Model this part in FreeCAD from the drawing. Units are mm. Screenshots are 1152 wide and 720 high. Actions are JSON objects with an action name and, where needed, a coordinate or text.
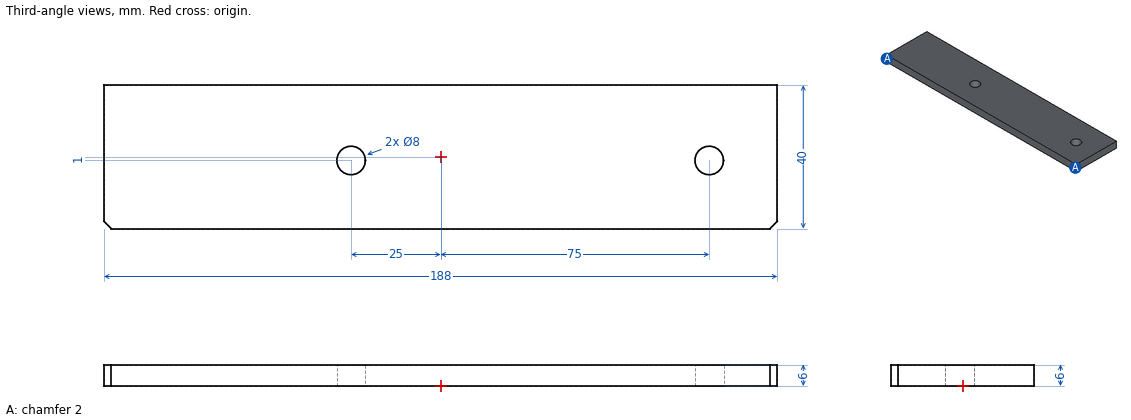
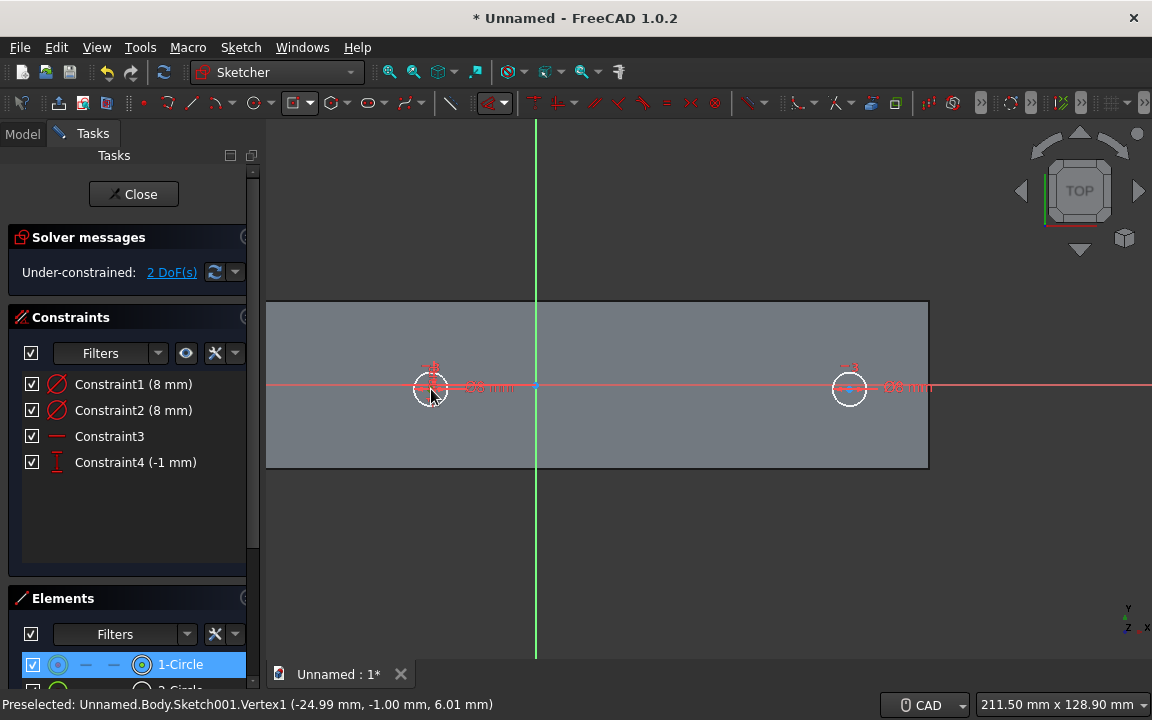
{"action": "left_click", "coordinate": [506, 104]}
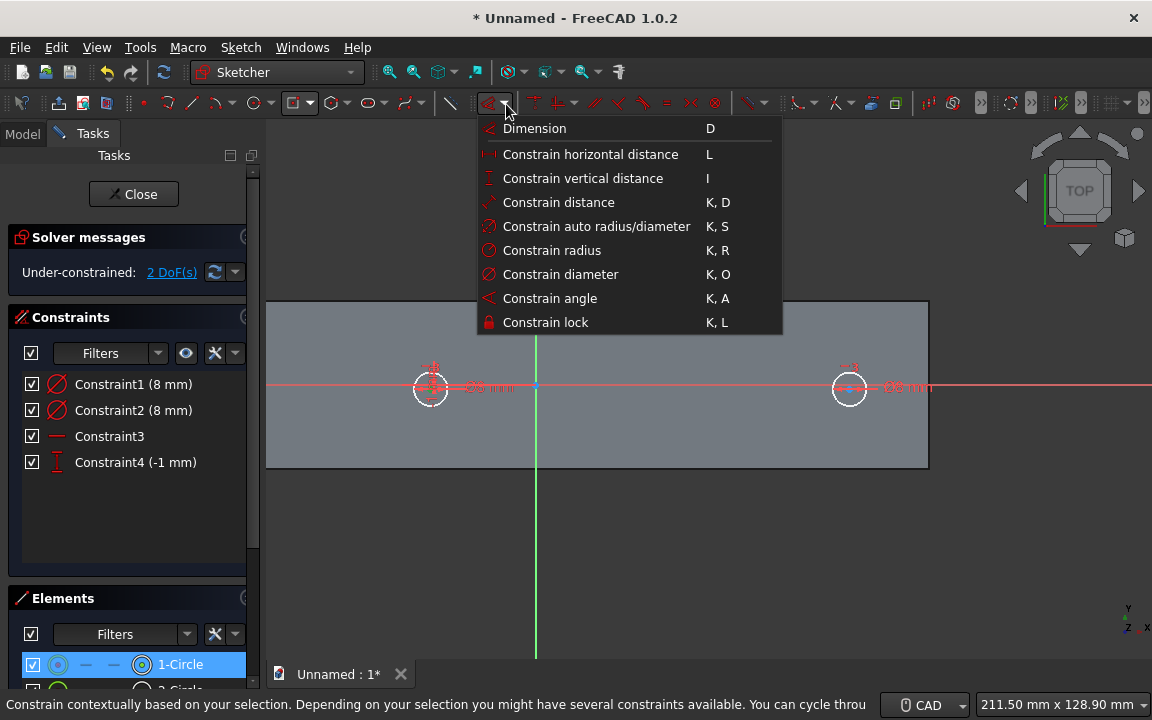
{"action": "left_click", "coordinate": [630, 154]}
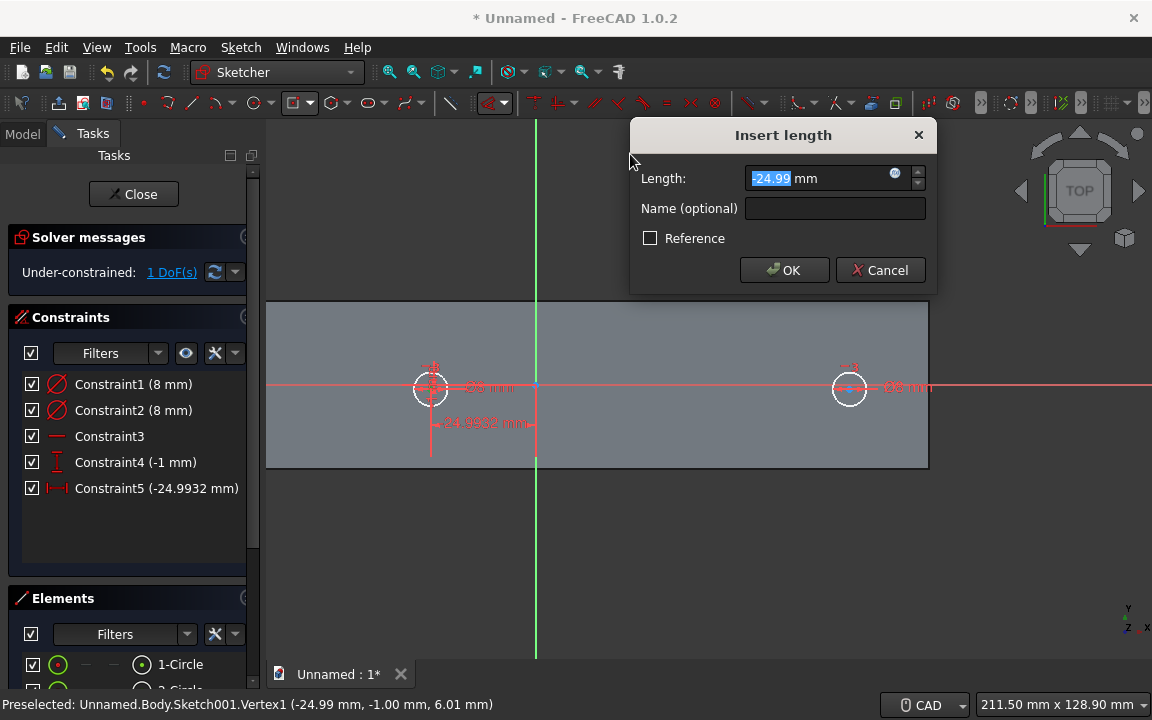
{"action": "type", "text": "-25"}
{"action": "key", "text": "Return"}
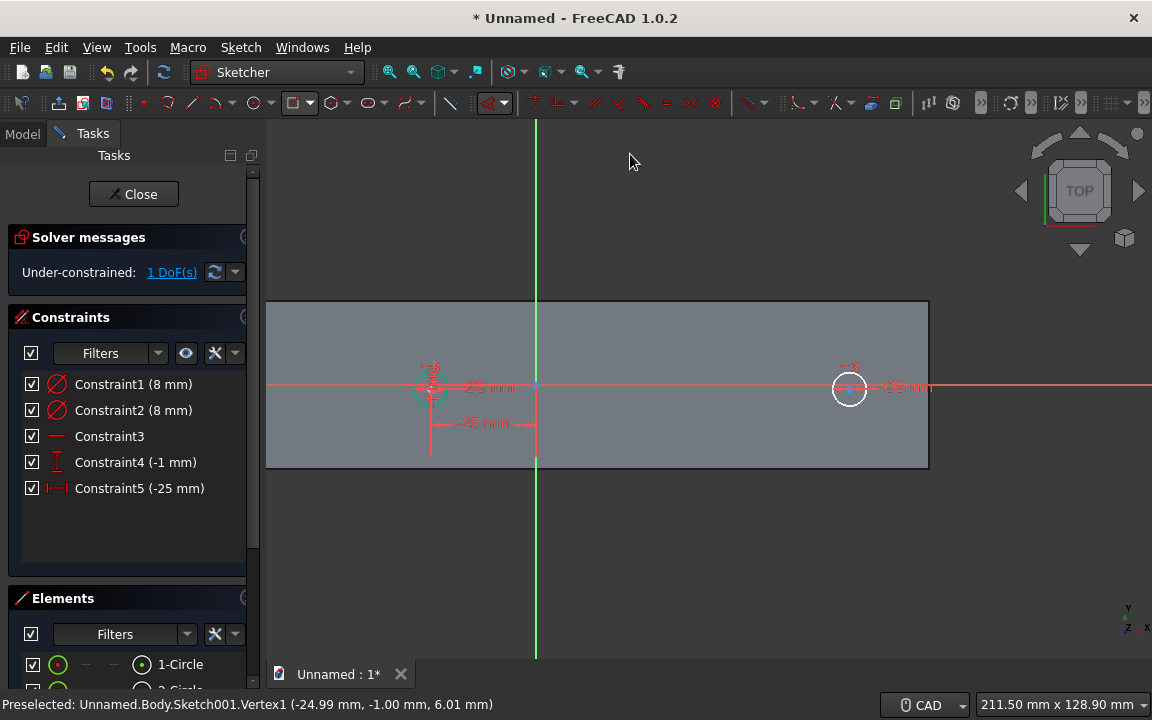
{"action": "left_click", "coordinate": [850, 389]}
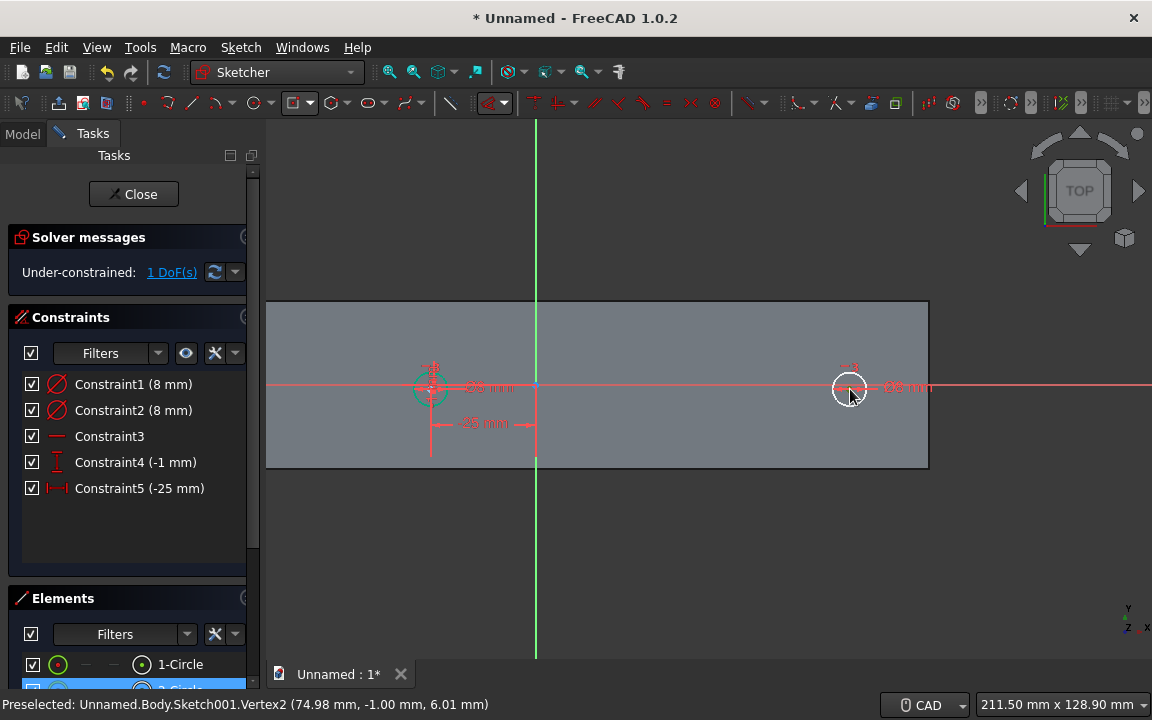
{"action": "left_click", "coordinate": [506, 104]}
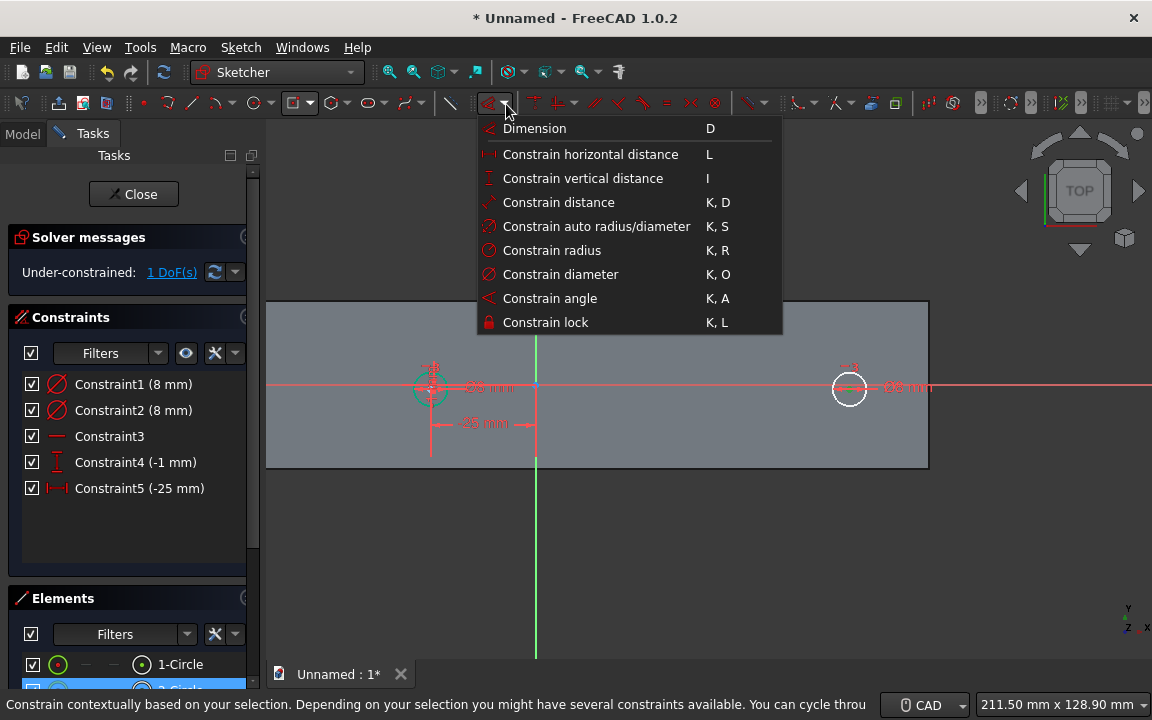
{"action": "left_click", "coordinate": [630, 154]}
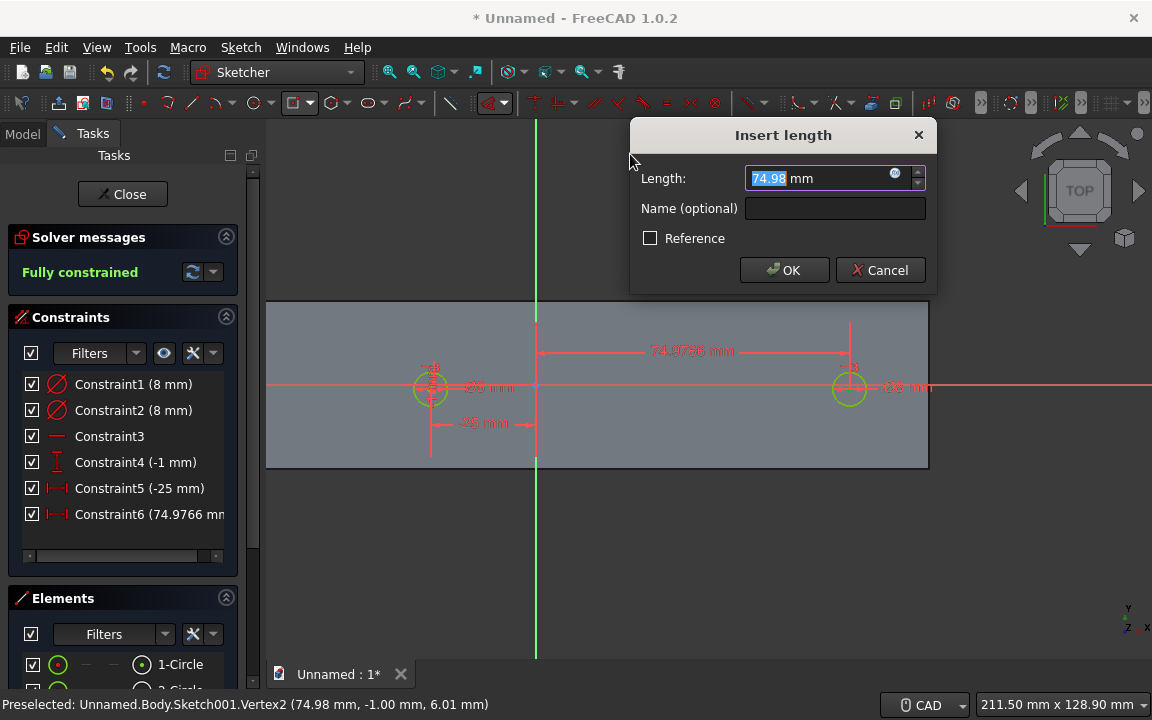
{"action": "type", "text": "75"}
{"action": "key", "text": "Return"}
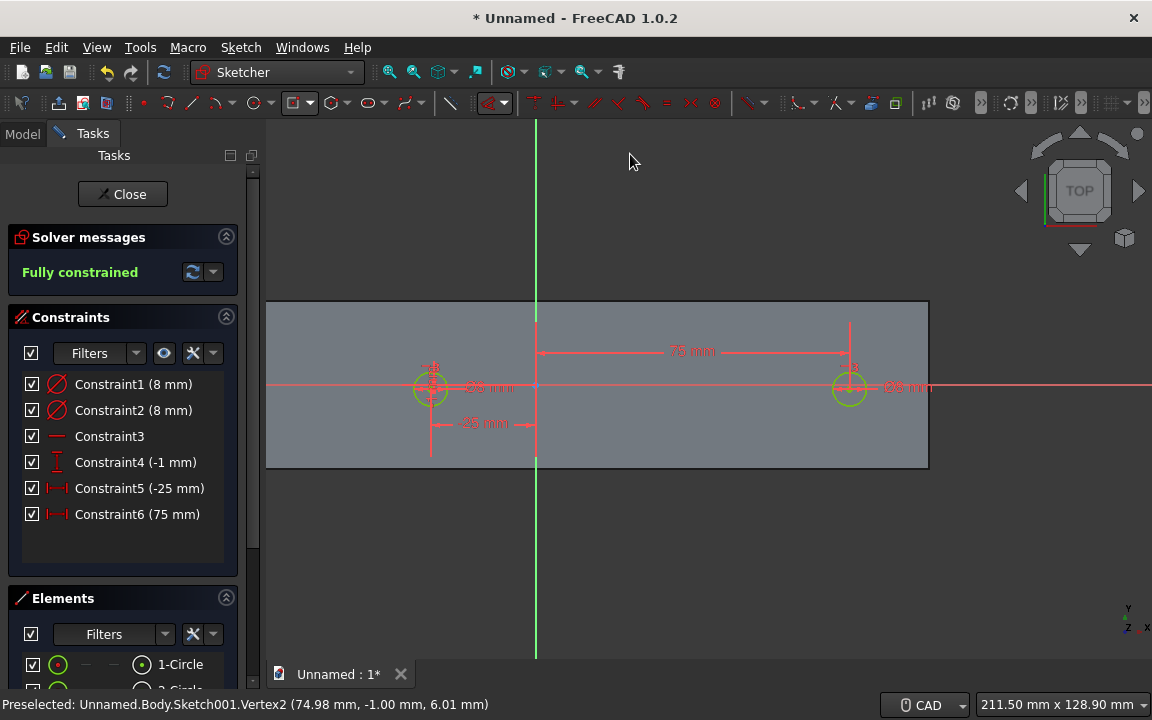
{"action": "left_click", "coordinate": [123, 194]}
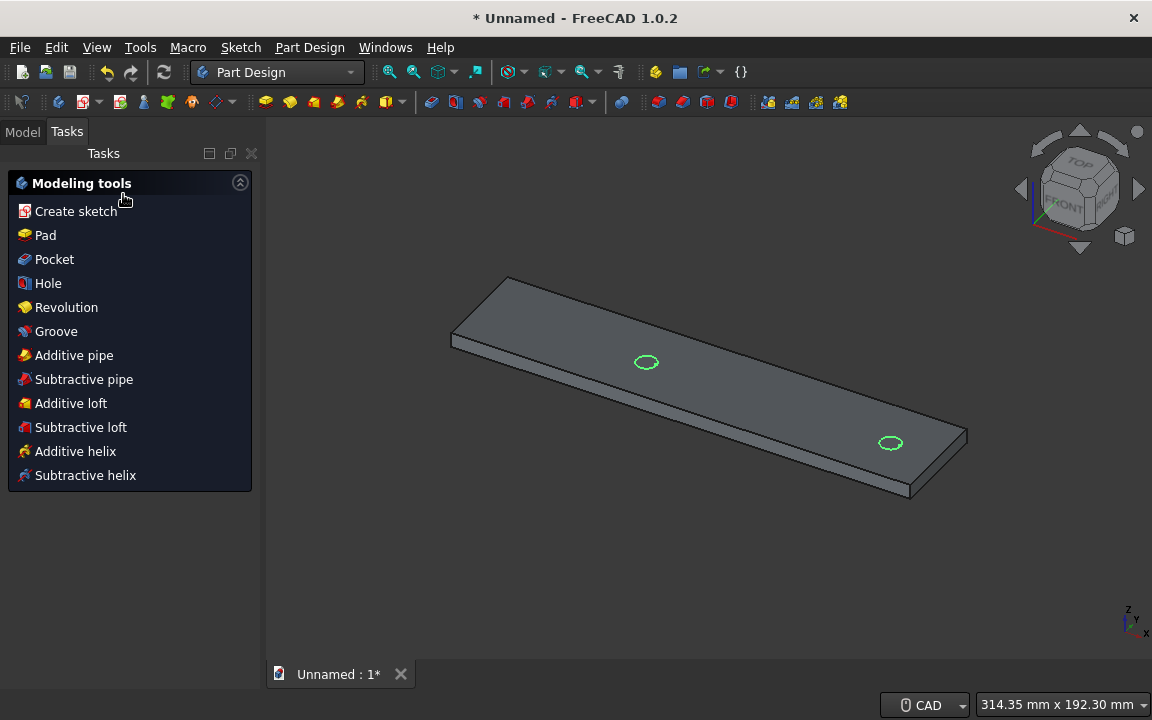
{"action": "left_click", "coordinate": [432, 102]}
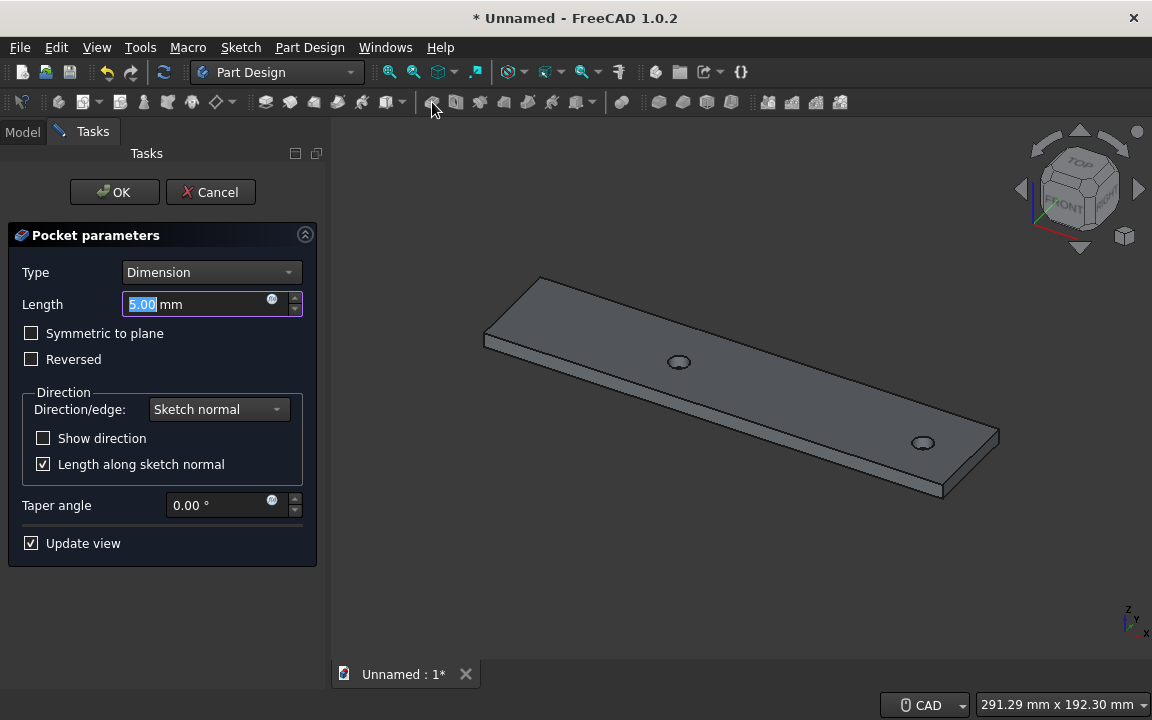
{"action": "type", "text": "6"}
{"action": "key", "text": "Tab"}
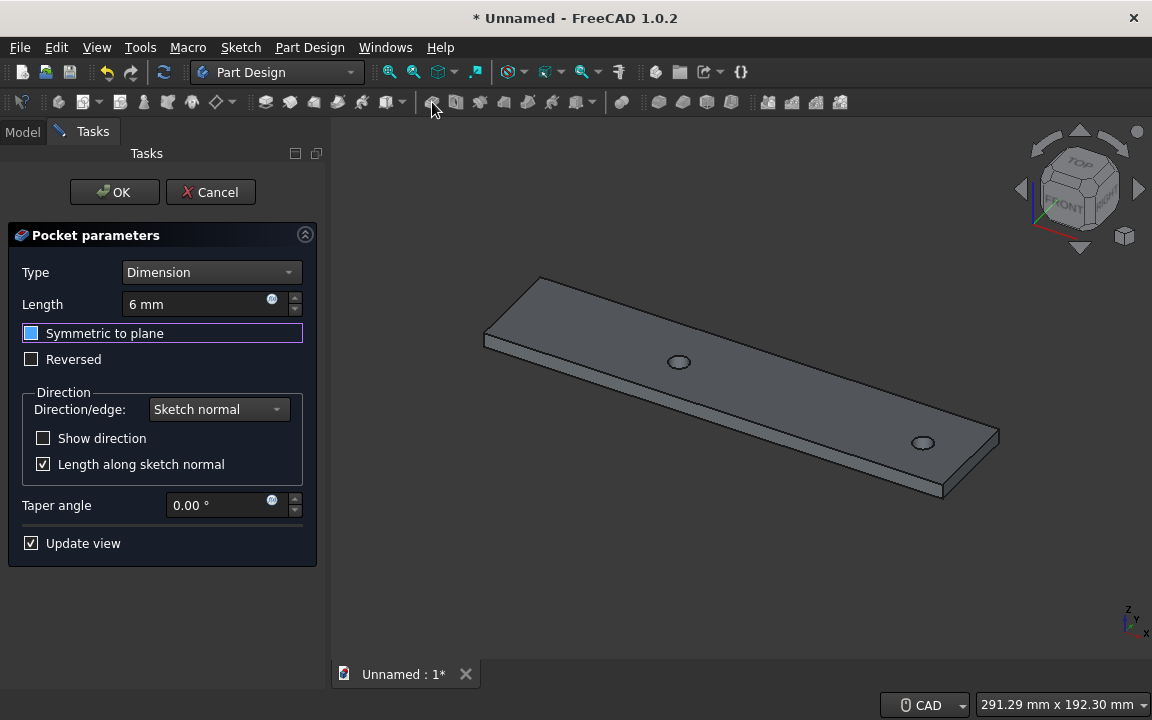
{"action": "left_click", "coordinate": [115, 192]}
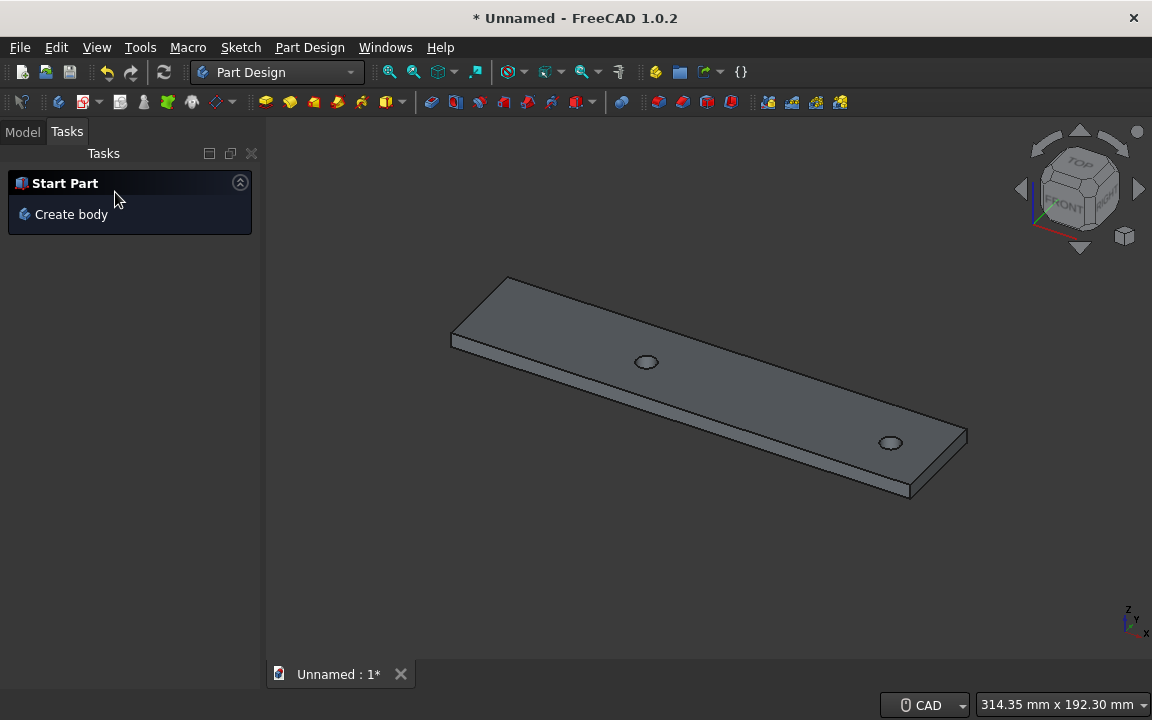
{"action": "left_click", "coordinate": [910, 491]}